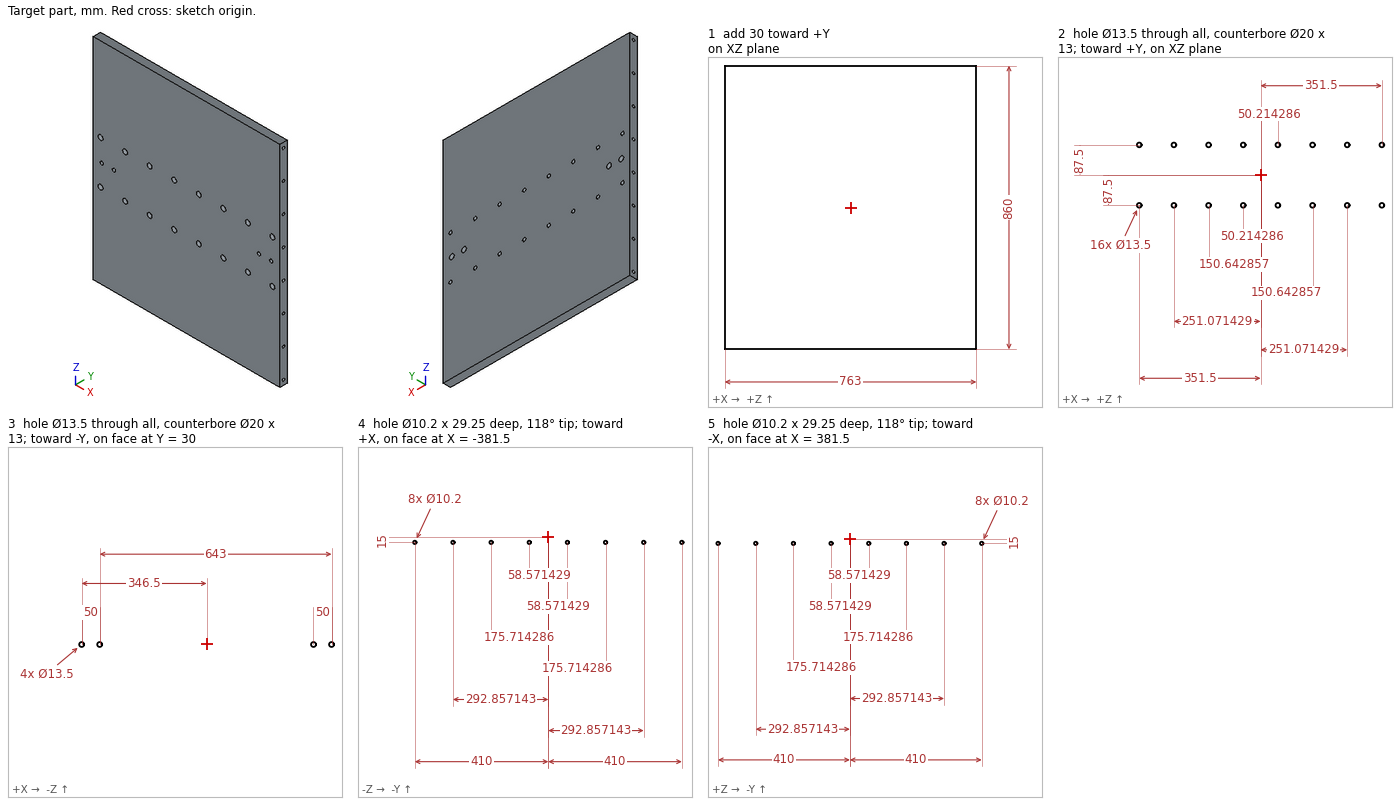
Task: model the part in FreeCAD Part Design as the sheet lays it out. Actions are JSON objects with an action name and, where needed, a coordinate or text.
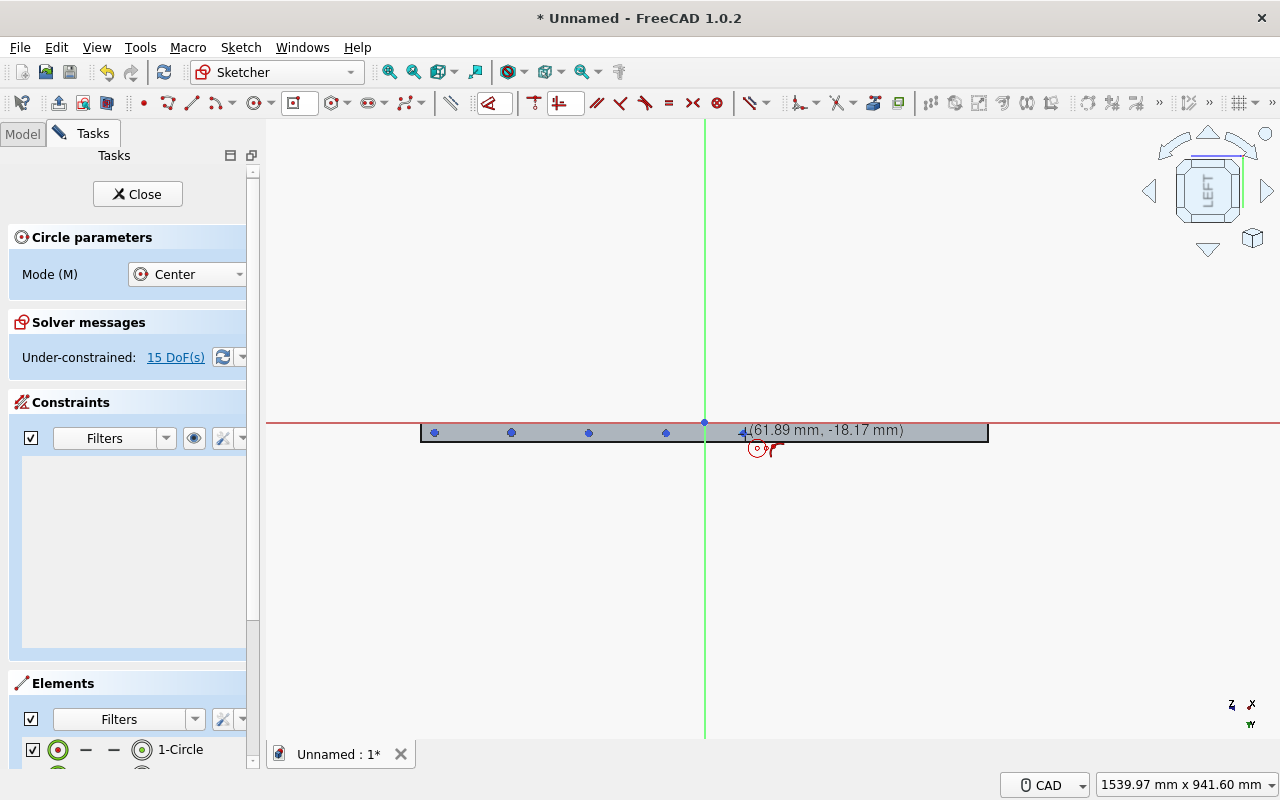
{"action": "scroll", "coordinate": [820, 433], "scroll_direction": "up", "scroll_amount": 10}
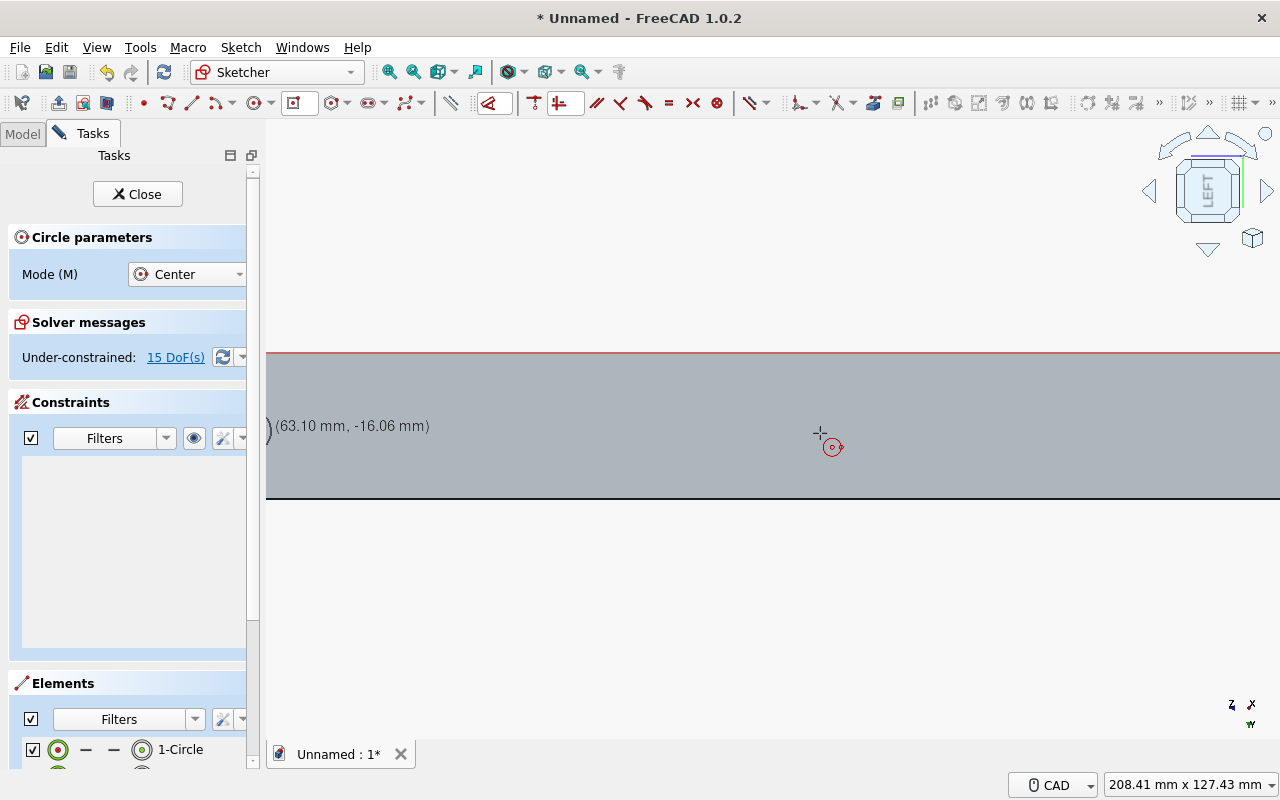
{"action": "scroll", "coordinate": [820, 433], "scroll_direction": "down", "scroll_amount": 10}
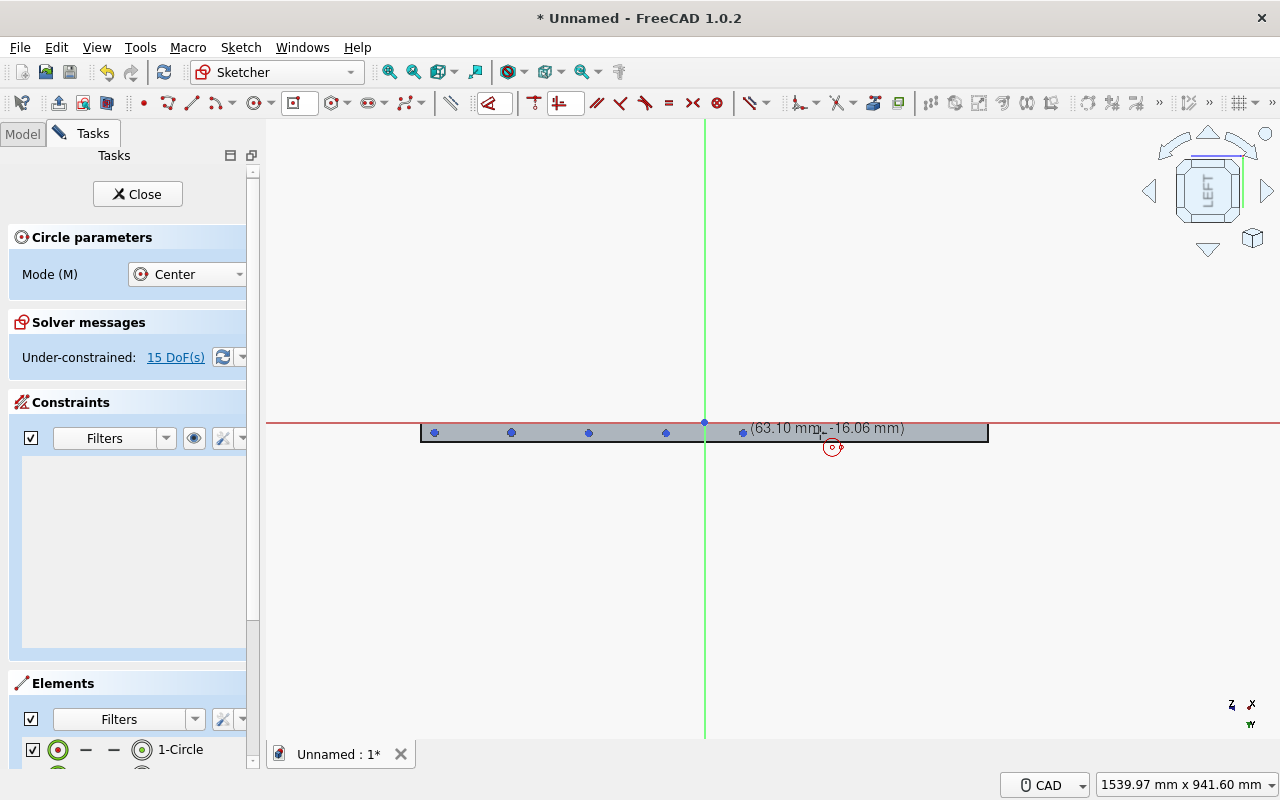
{"action": "scroll", "coordinate": [820, 433], "scroll_direction": "up", "scroll_amount": 3}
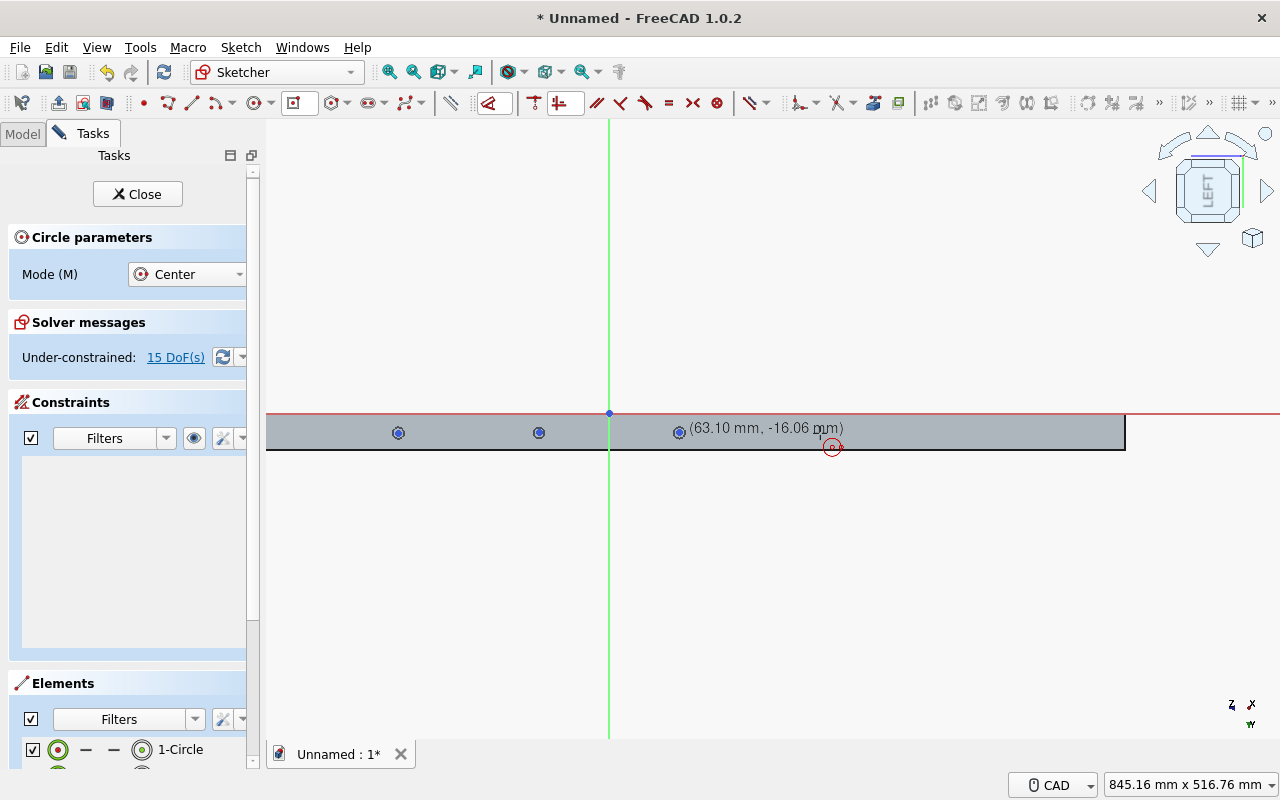
{"action": "left_click", "coordinate": [820, 432]}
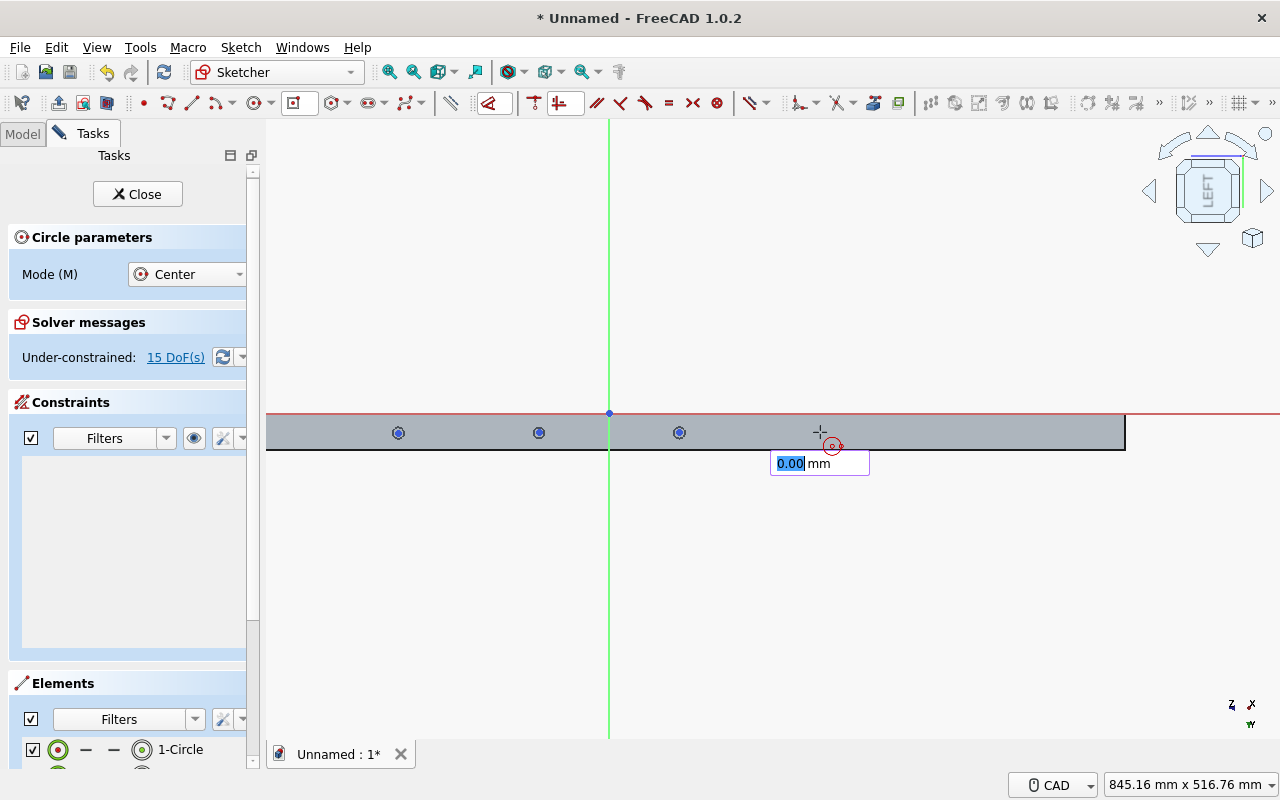
{"action": "scroll", "coordinate": [824, 436], "scroll_direction": "up", "scroll_amount": 5}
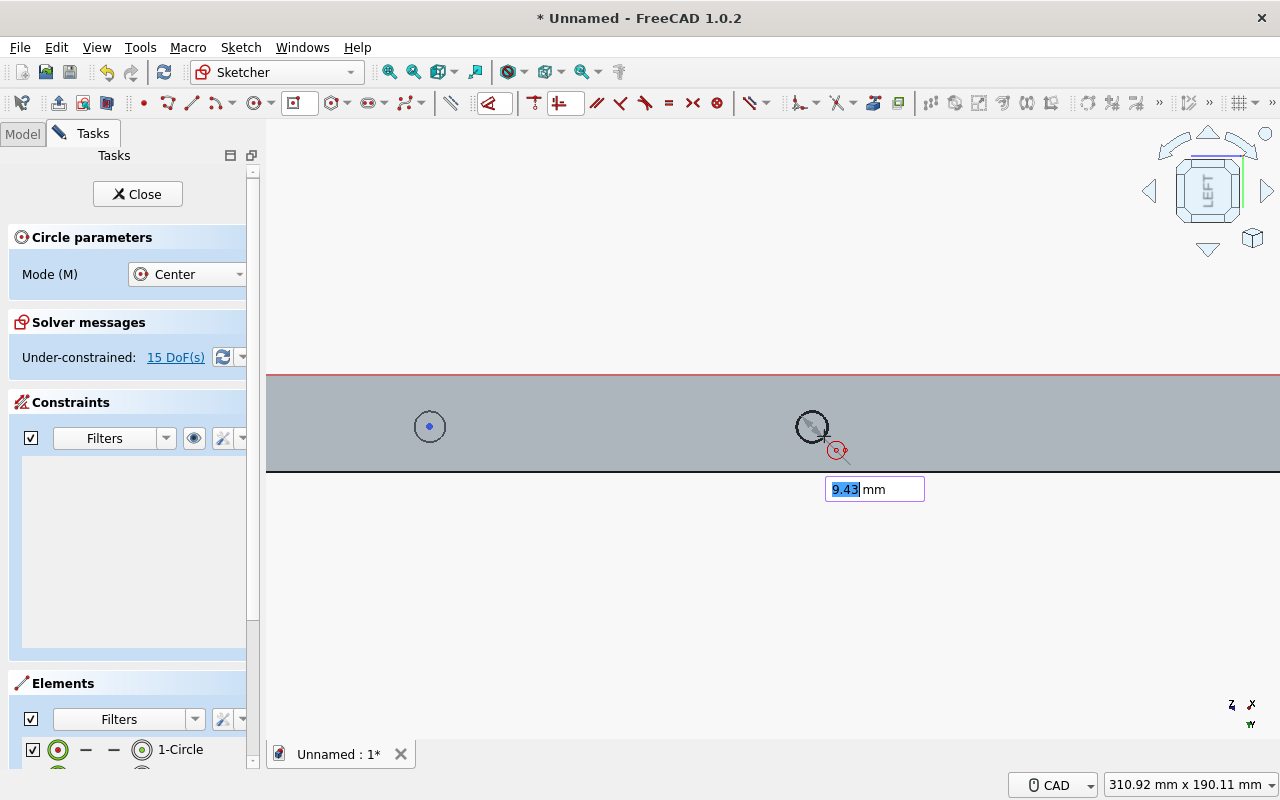
{"action": "left_click", "coordinate": [824, 435]}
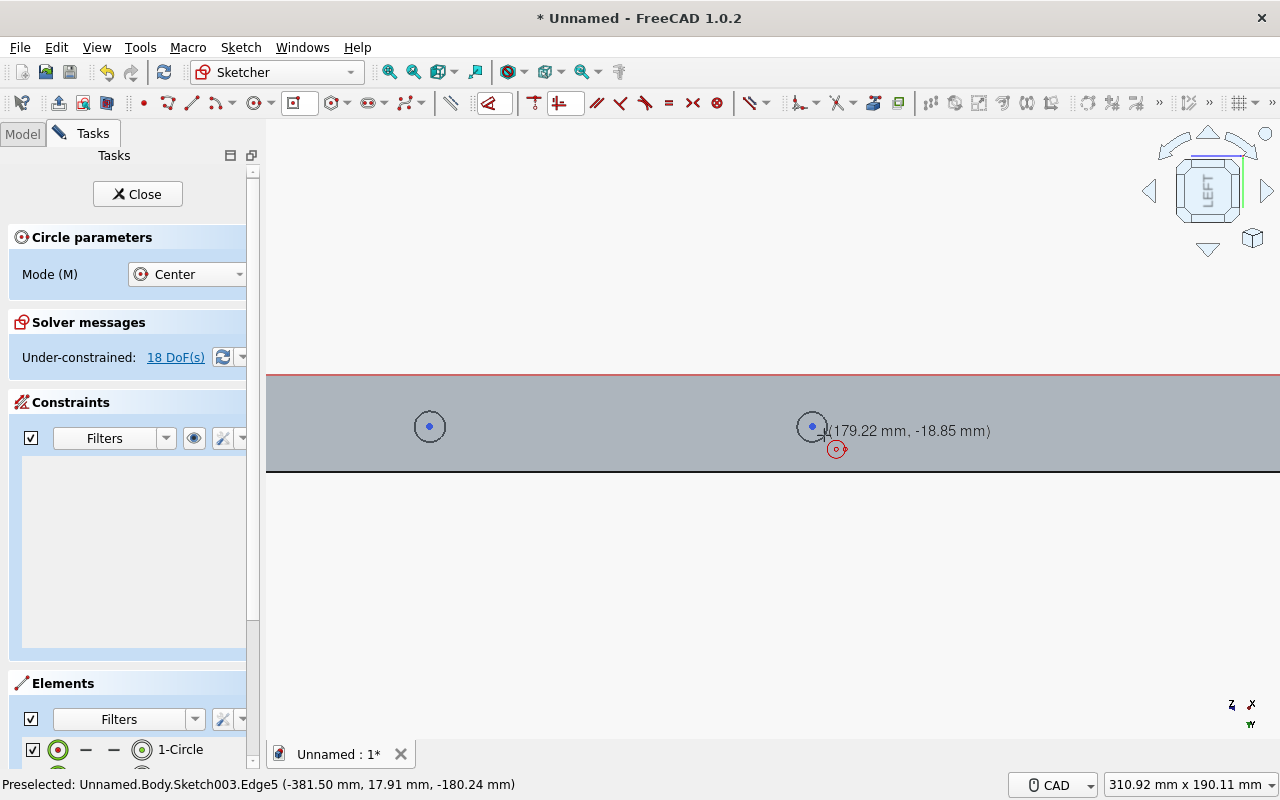
{"action": "scroll", "coordinate": [822, 434], "scroll_direction": "down", "scroll_amount": 8}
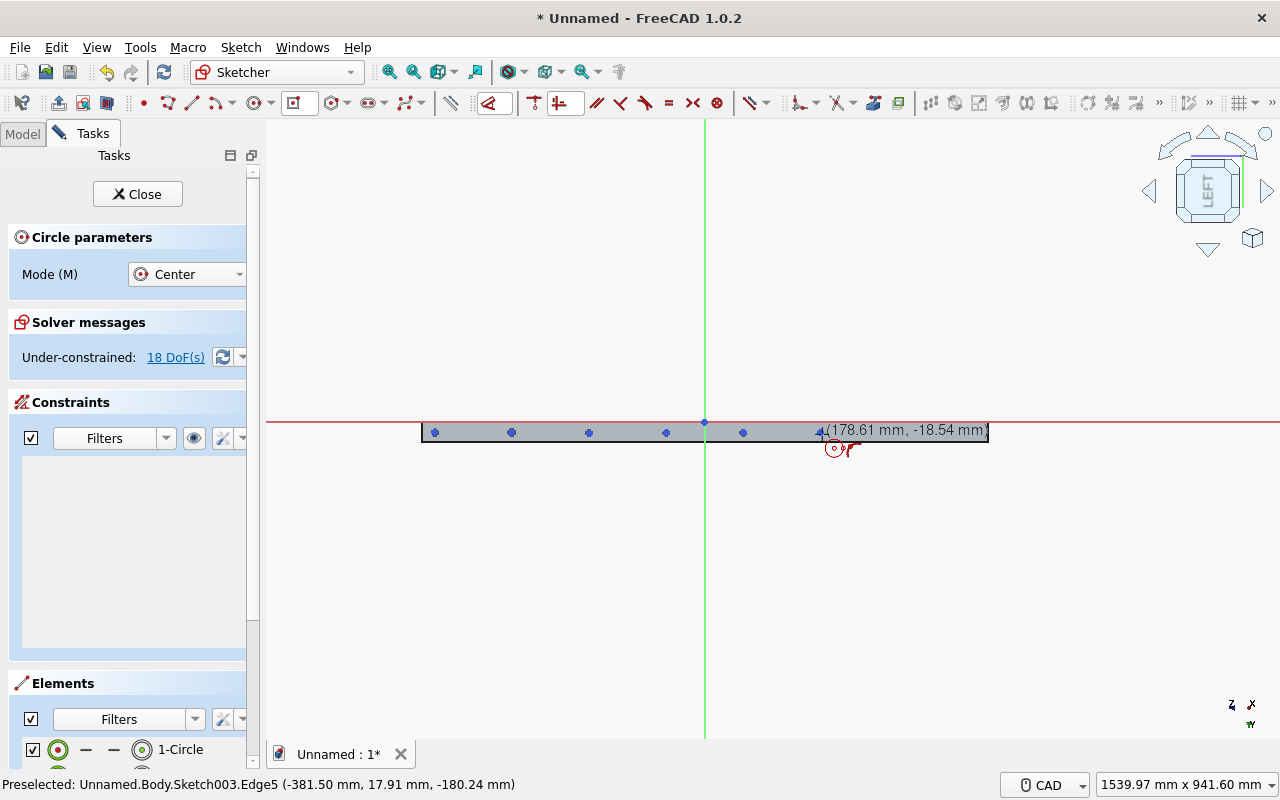
{"action": "scroll", "coordinate": [898, 432], "scroll_direction": "up", "scroll_amount": 10}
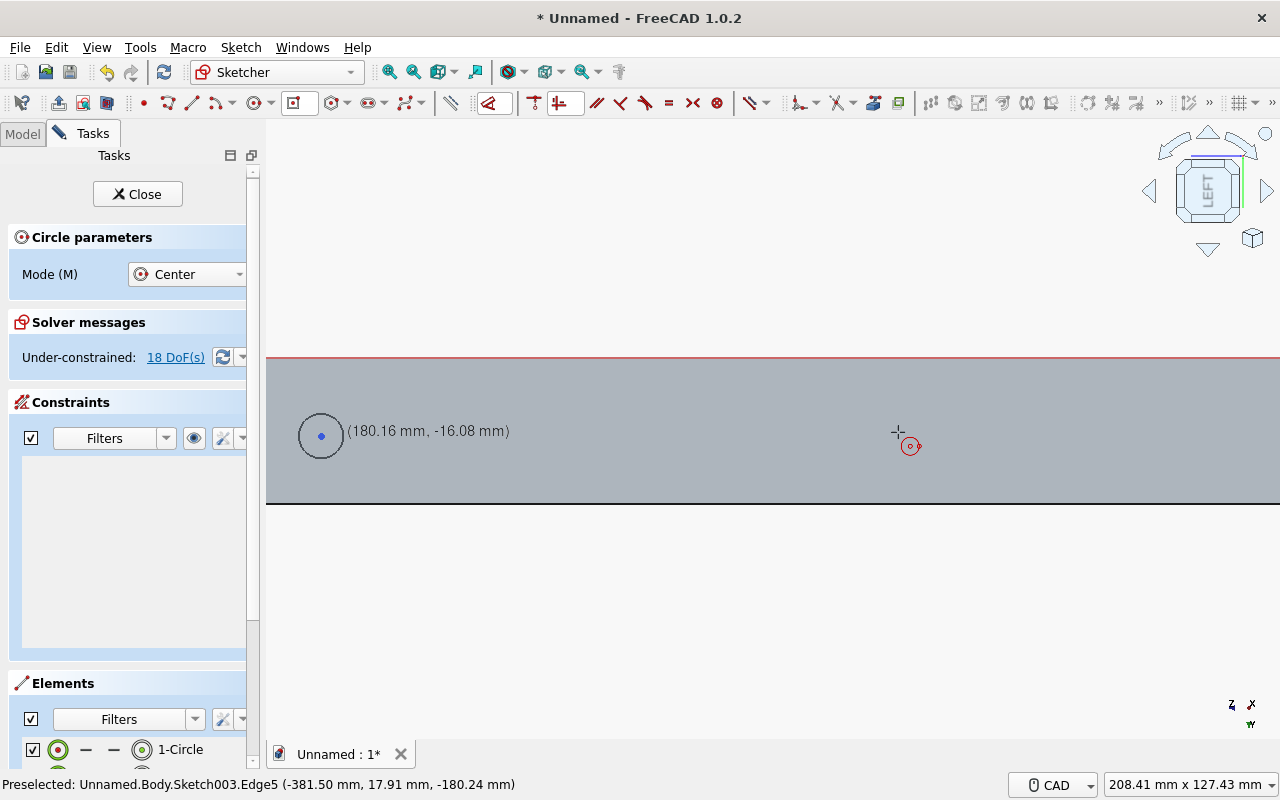
{"action": "scroll", "coordinate": [898, 432], "scroll_direction": "down", "scroll_amount": 10}